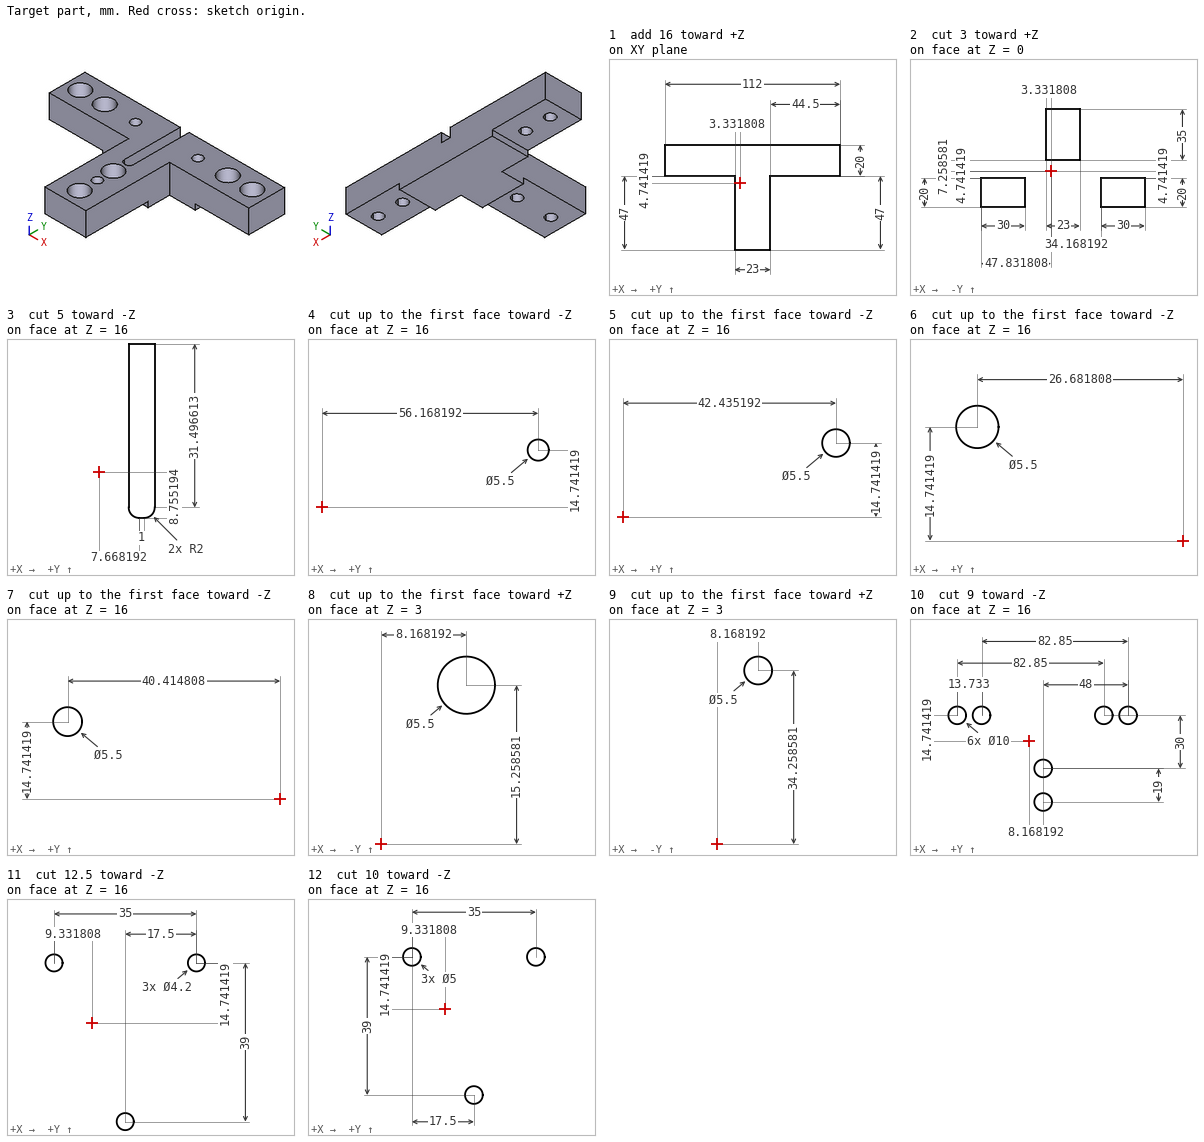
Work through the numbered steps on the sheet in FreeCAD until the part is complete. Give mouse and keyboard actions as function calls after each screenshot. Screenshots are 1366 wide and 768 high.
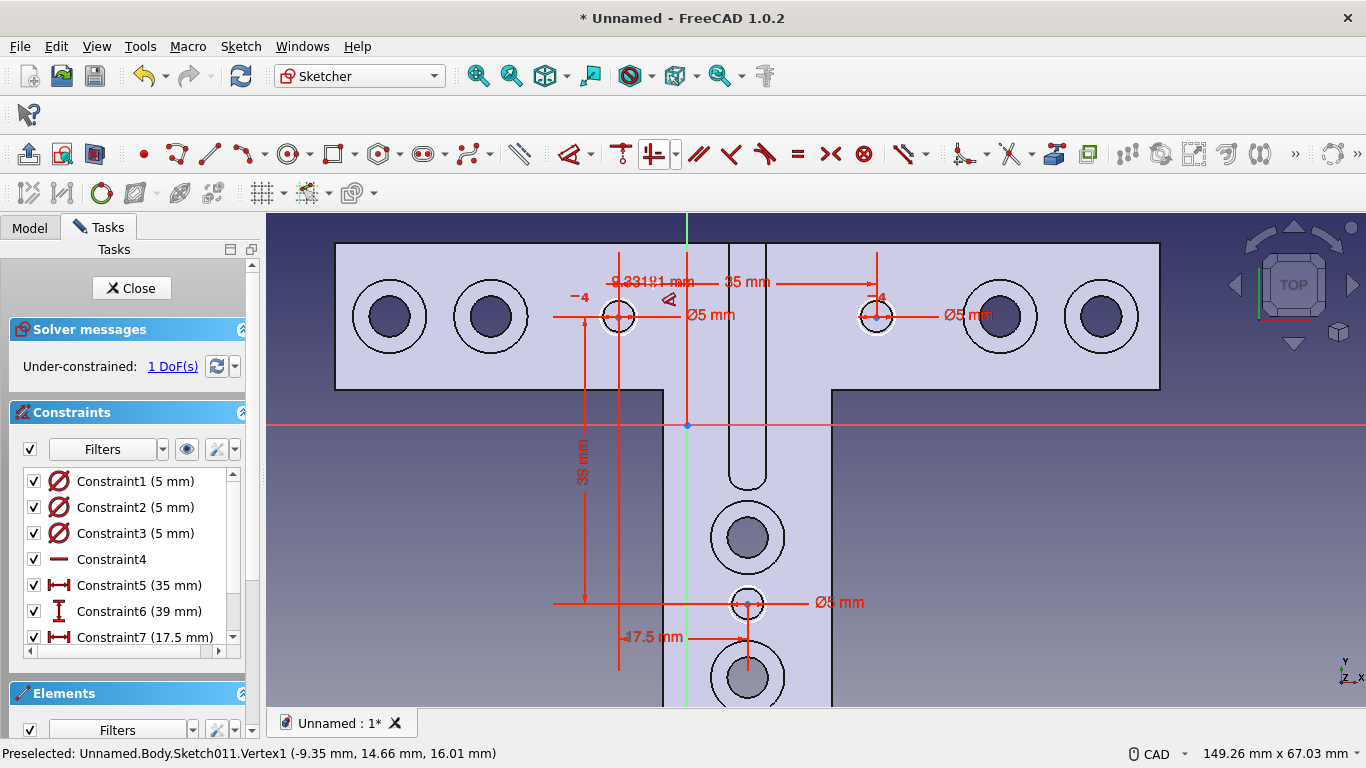
click(619, 317)
click(585, 371)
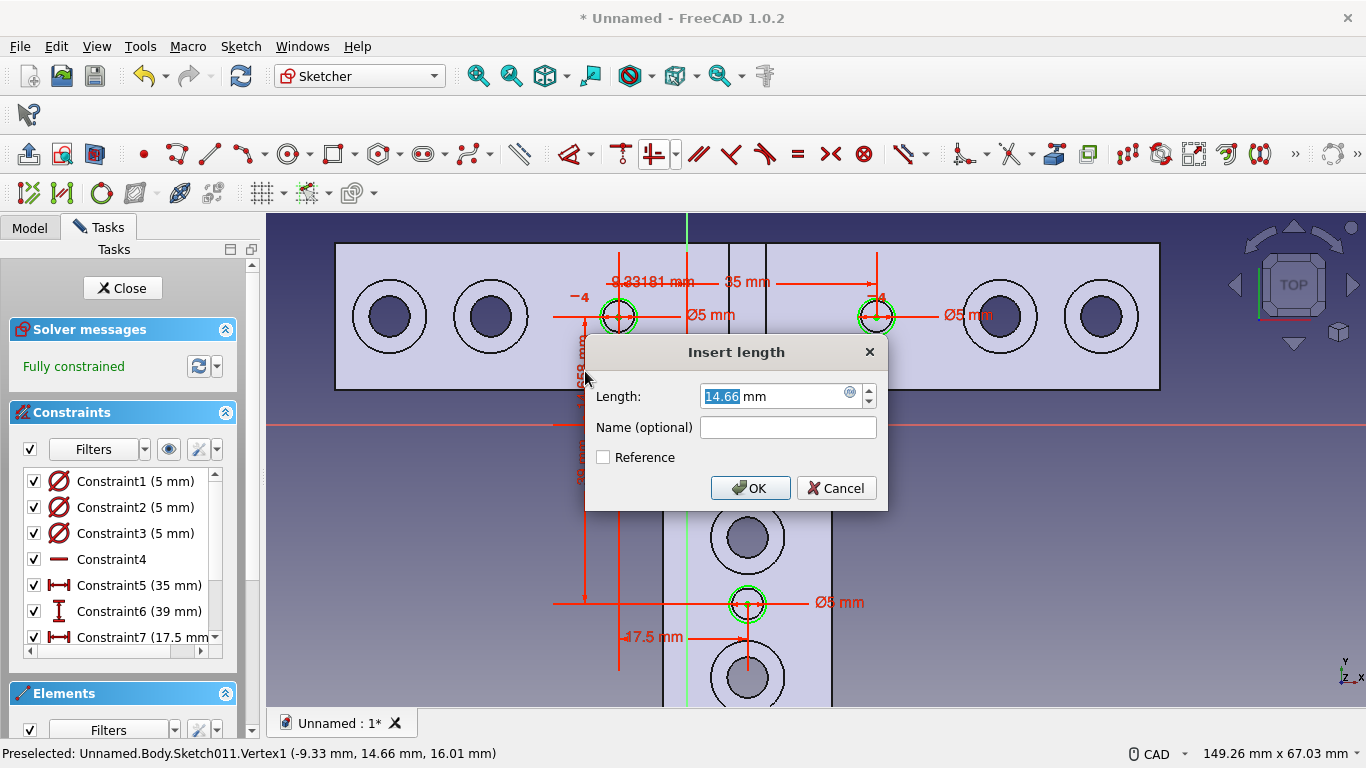
text(14.741419)
key(Return)
key(Escape)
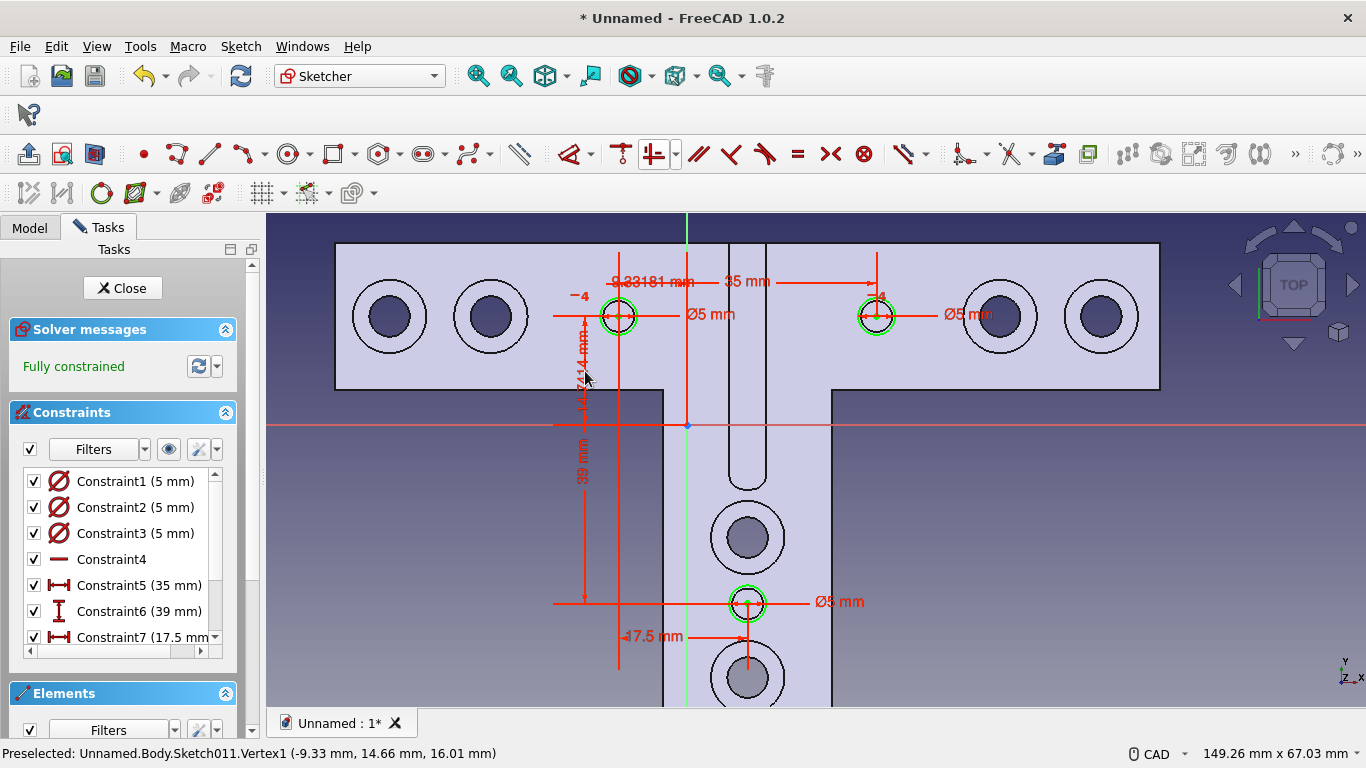
click(123, 288)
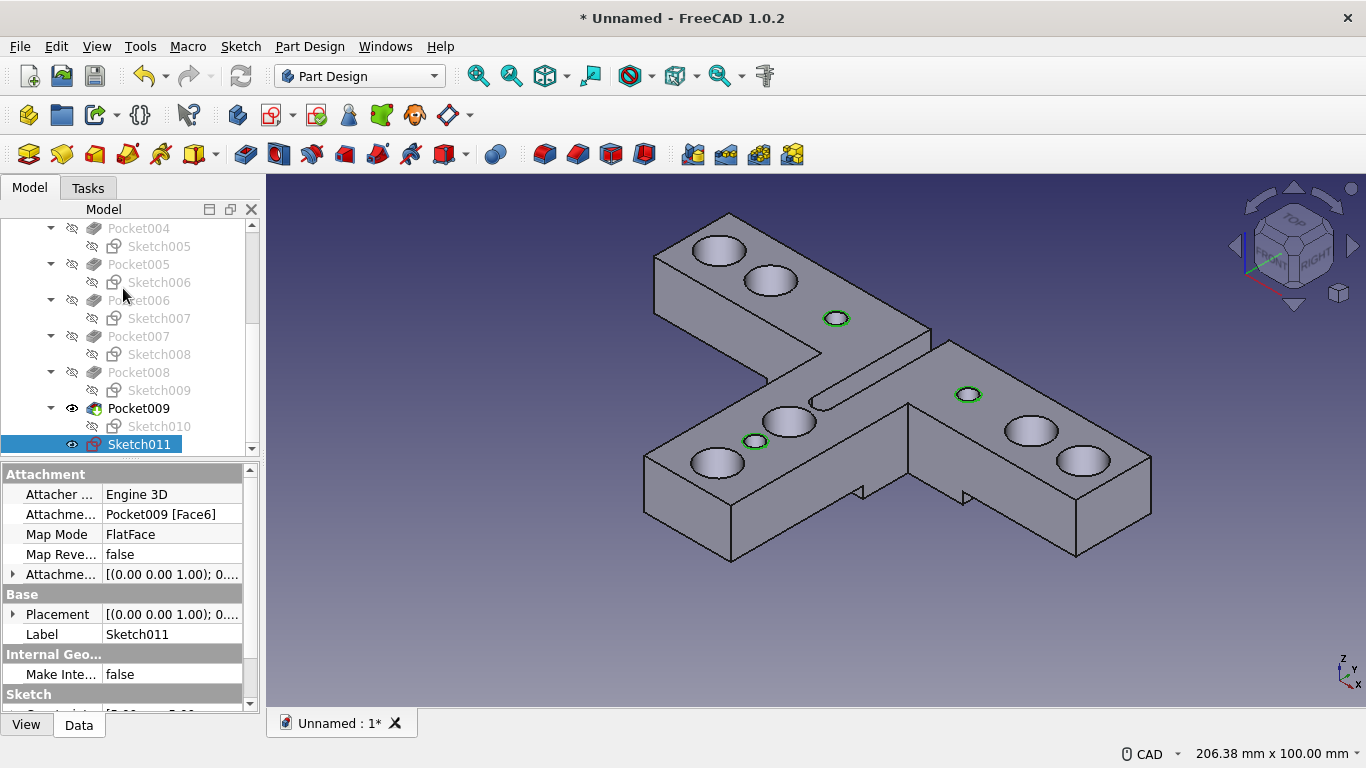
click(246, 154)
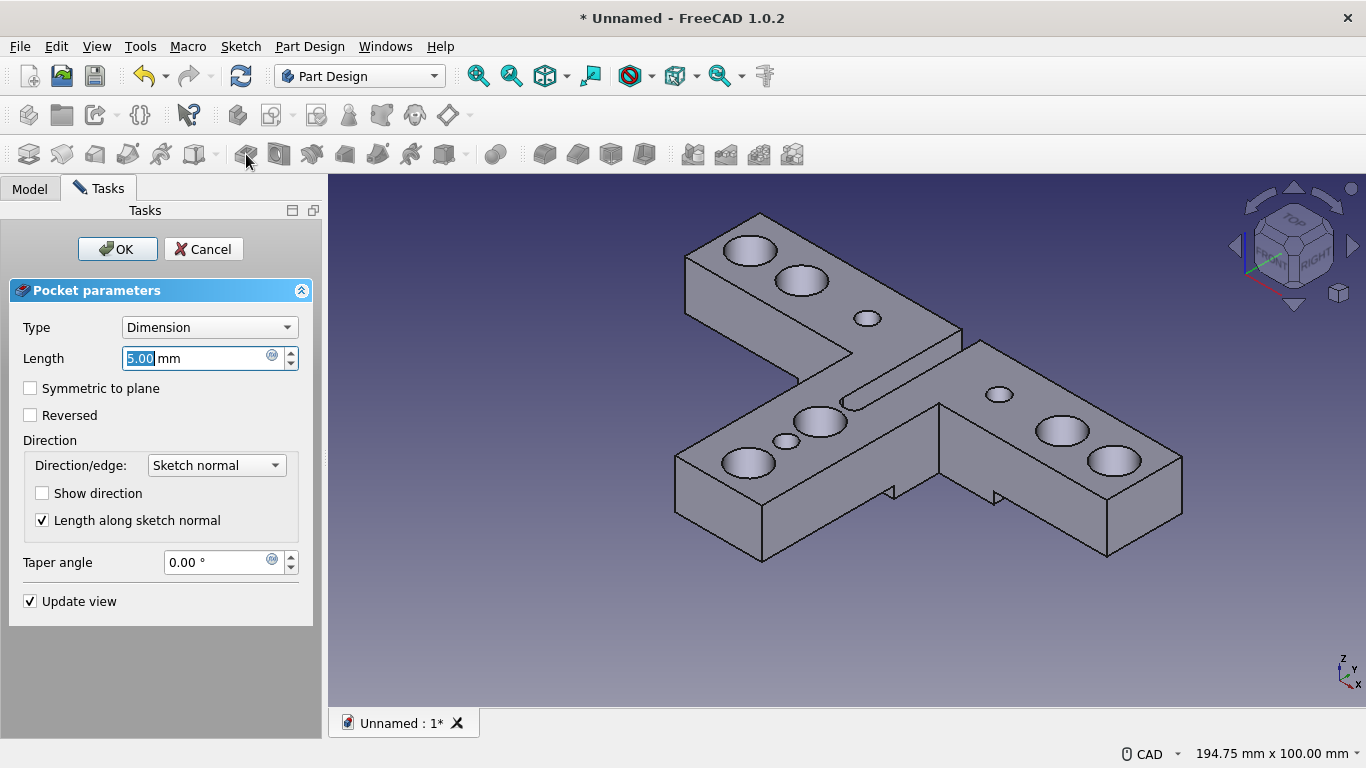
text(10)
key(Tab)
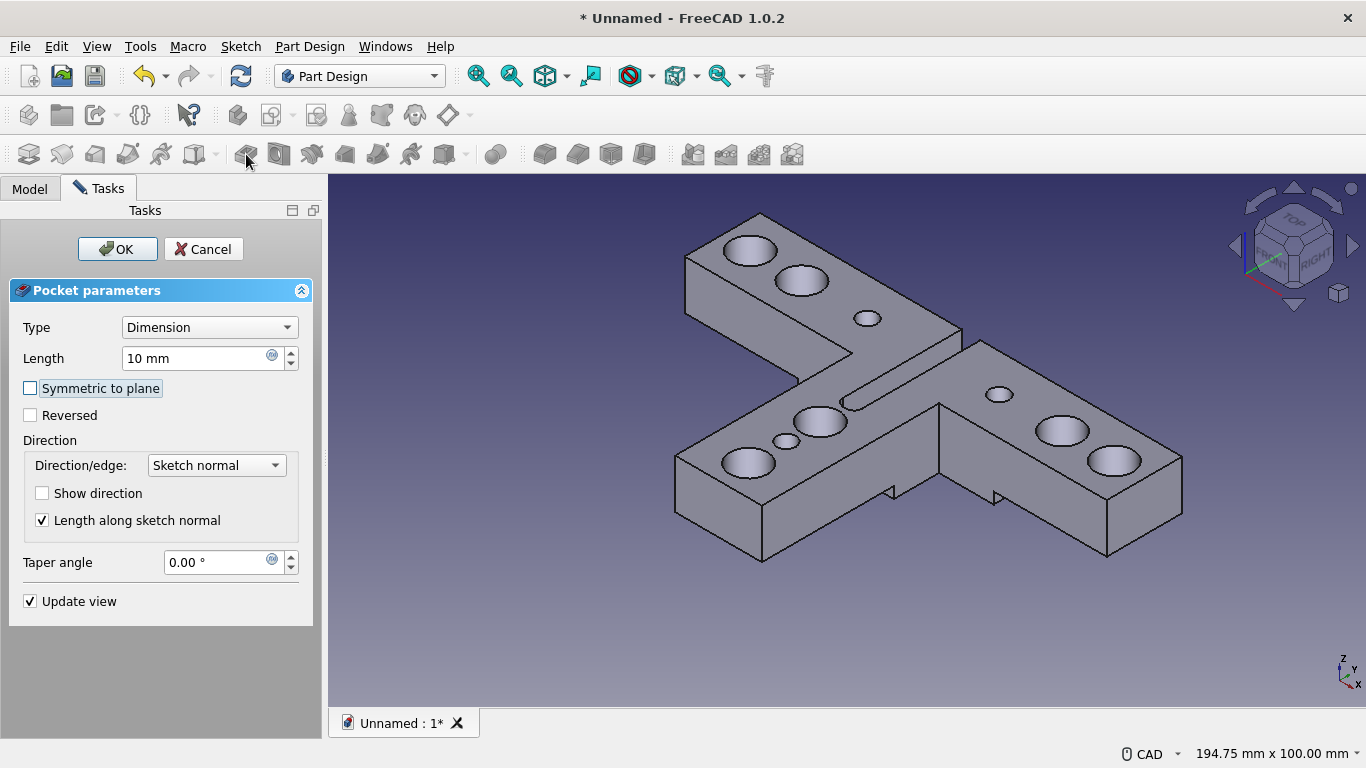
click(118, 249)